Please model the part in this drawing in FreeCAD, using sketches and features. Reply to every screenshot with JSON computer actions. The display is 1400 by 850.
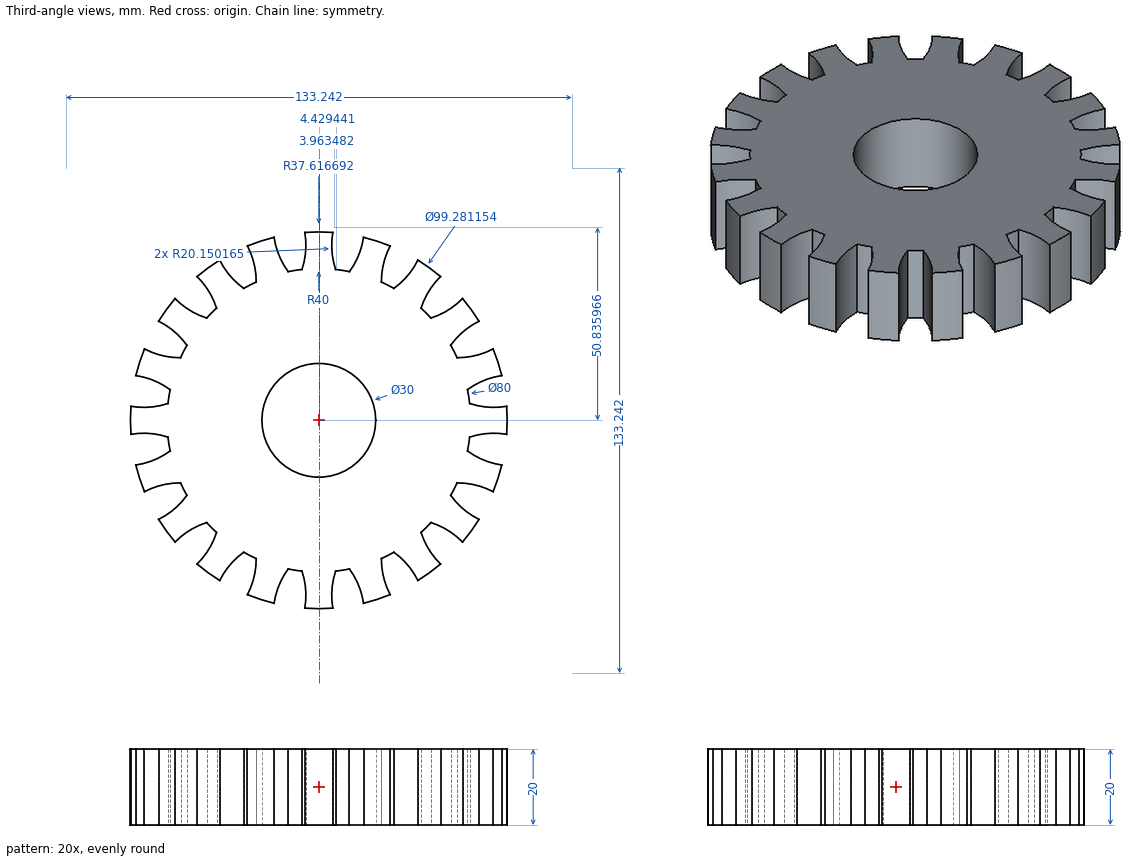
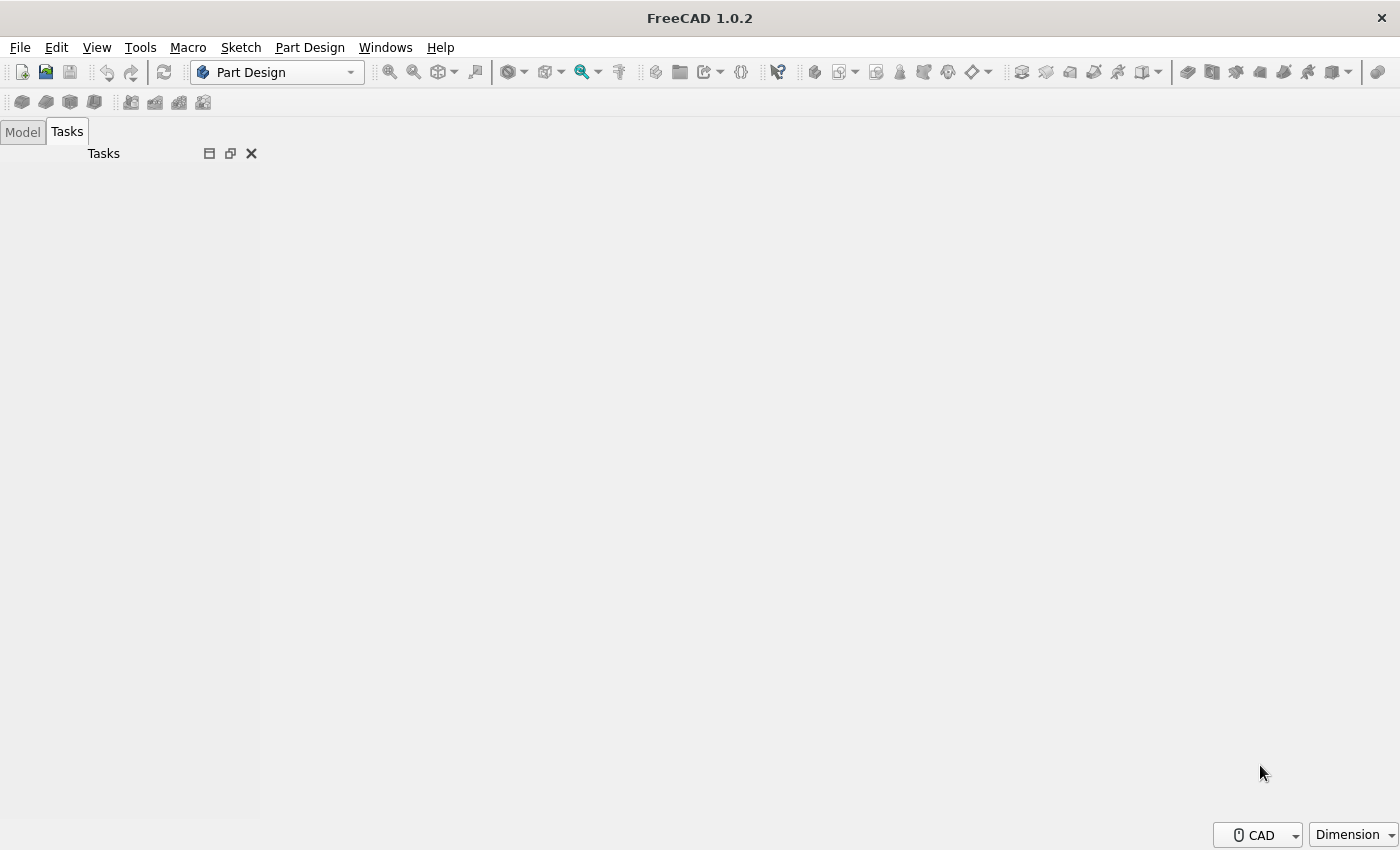
{"action": "left_click", "coordinate": [22, 72]}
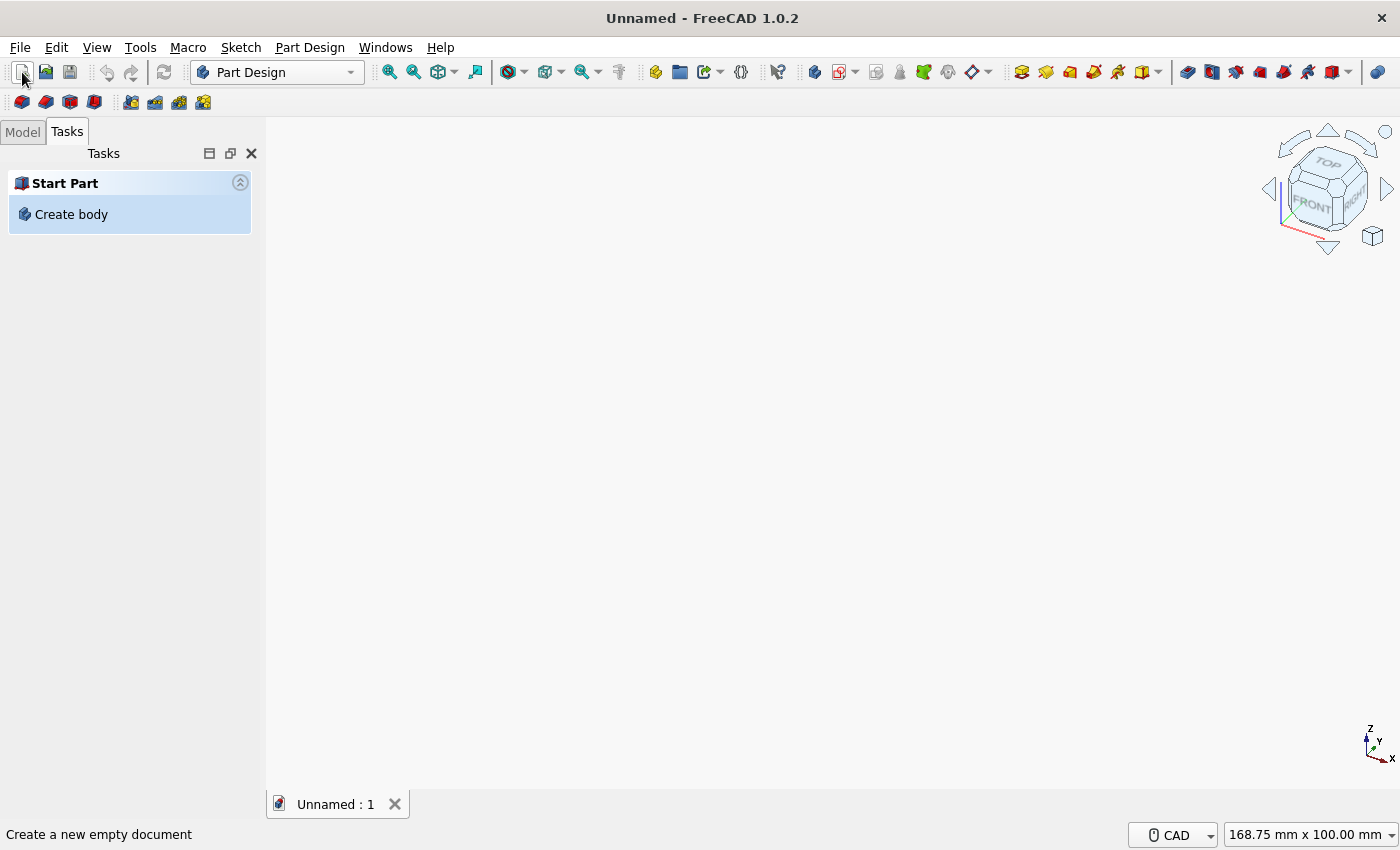
{"action": "left_click", "coordinate": [840, 72]}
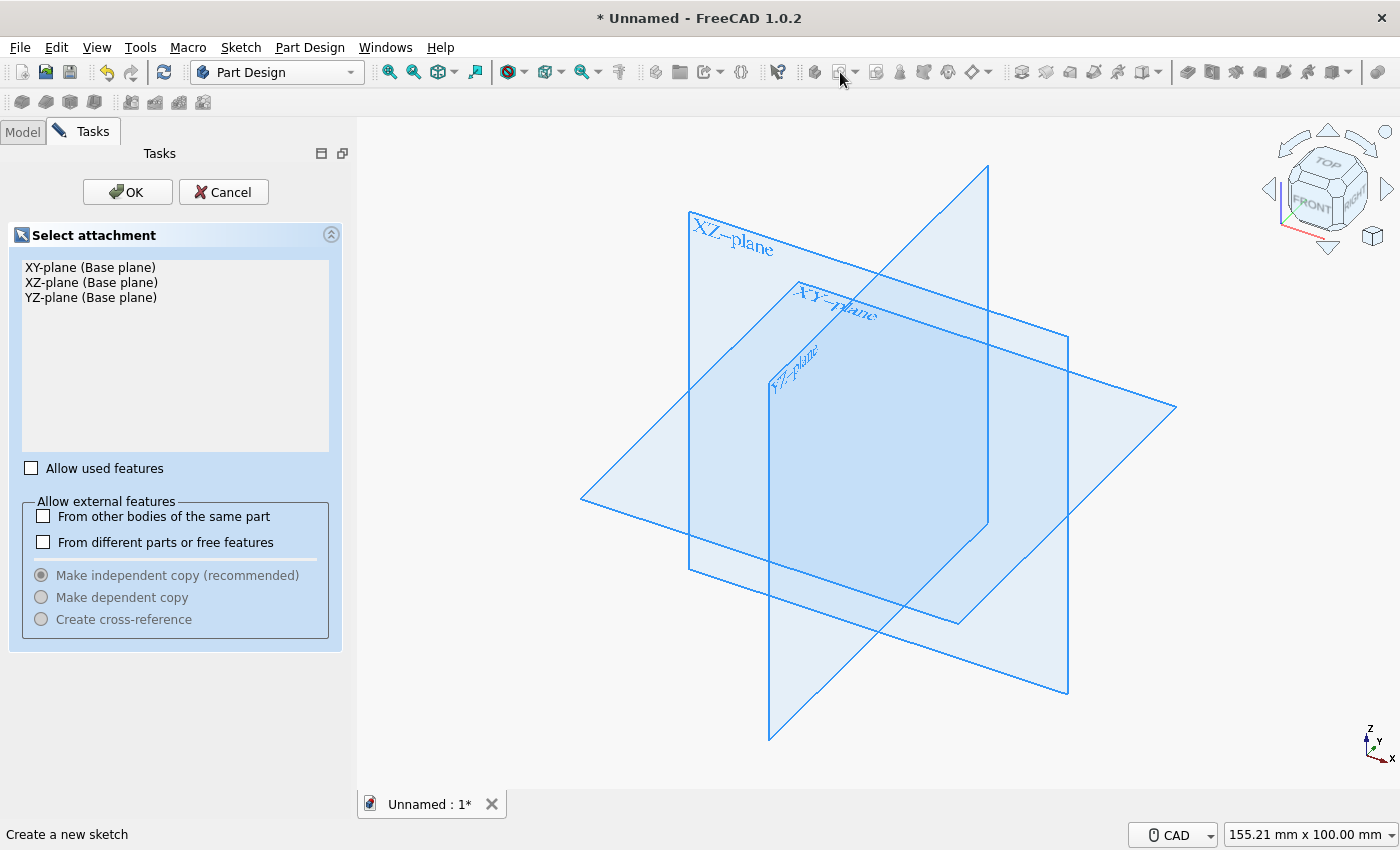
{"action": "left_click", "coordinate": [82, 268]}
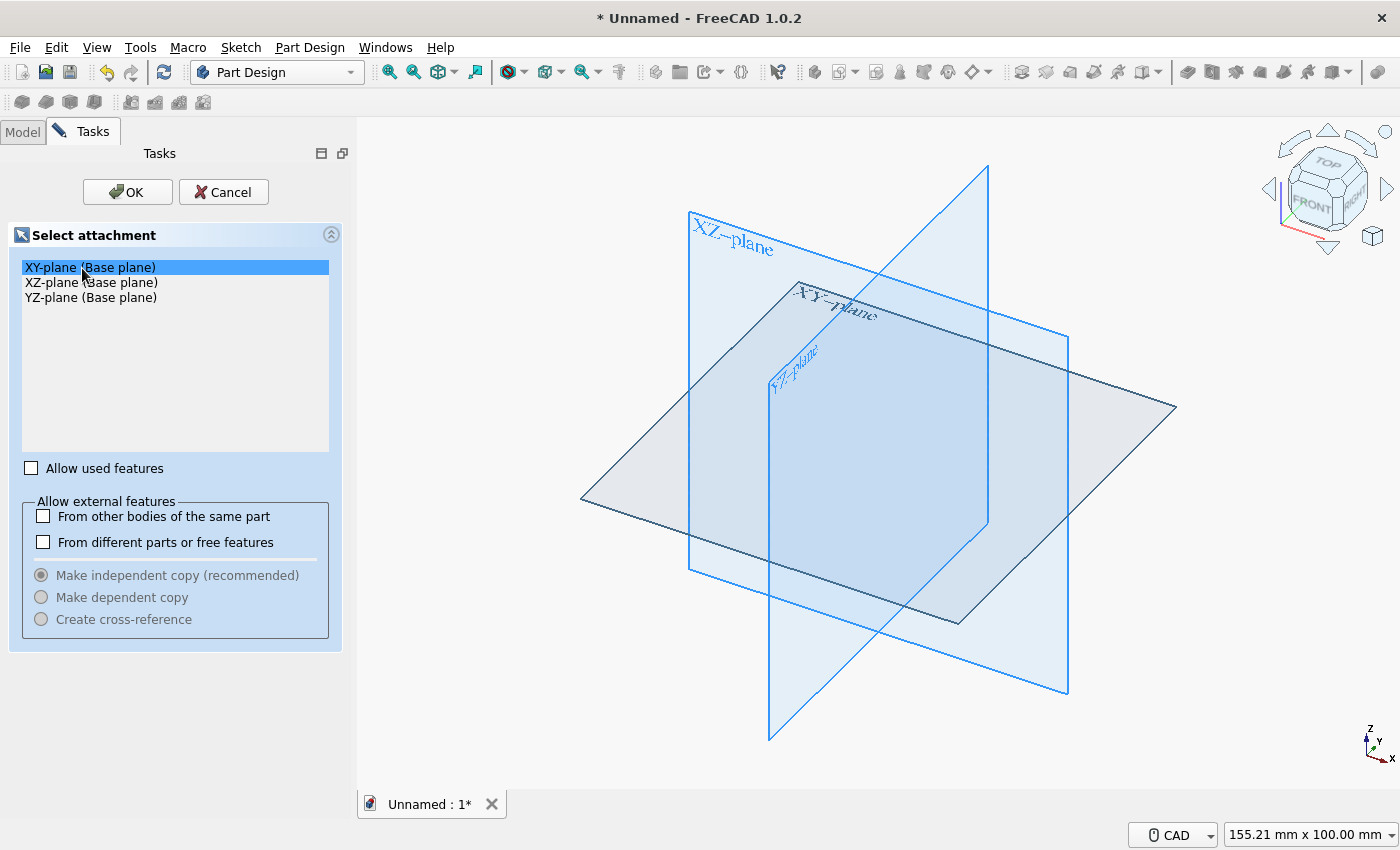
{"action": "left_click", "coordinate": [128, 192]}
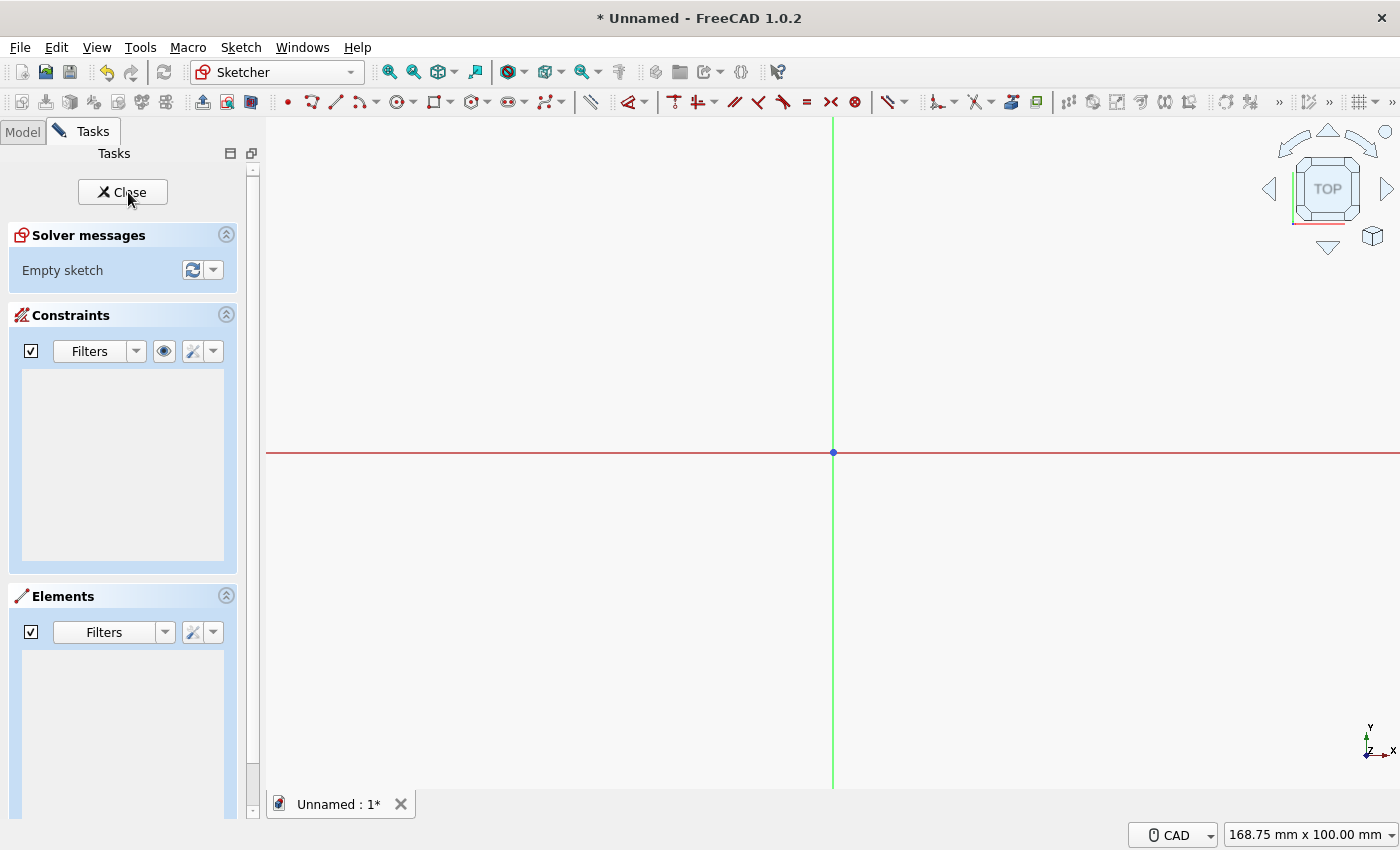
{"action": "left_click", "coordinate": [398, 102]}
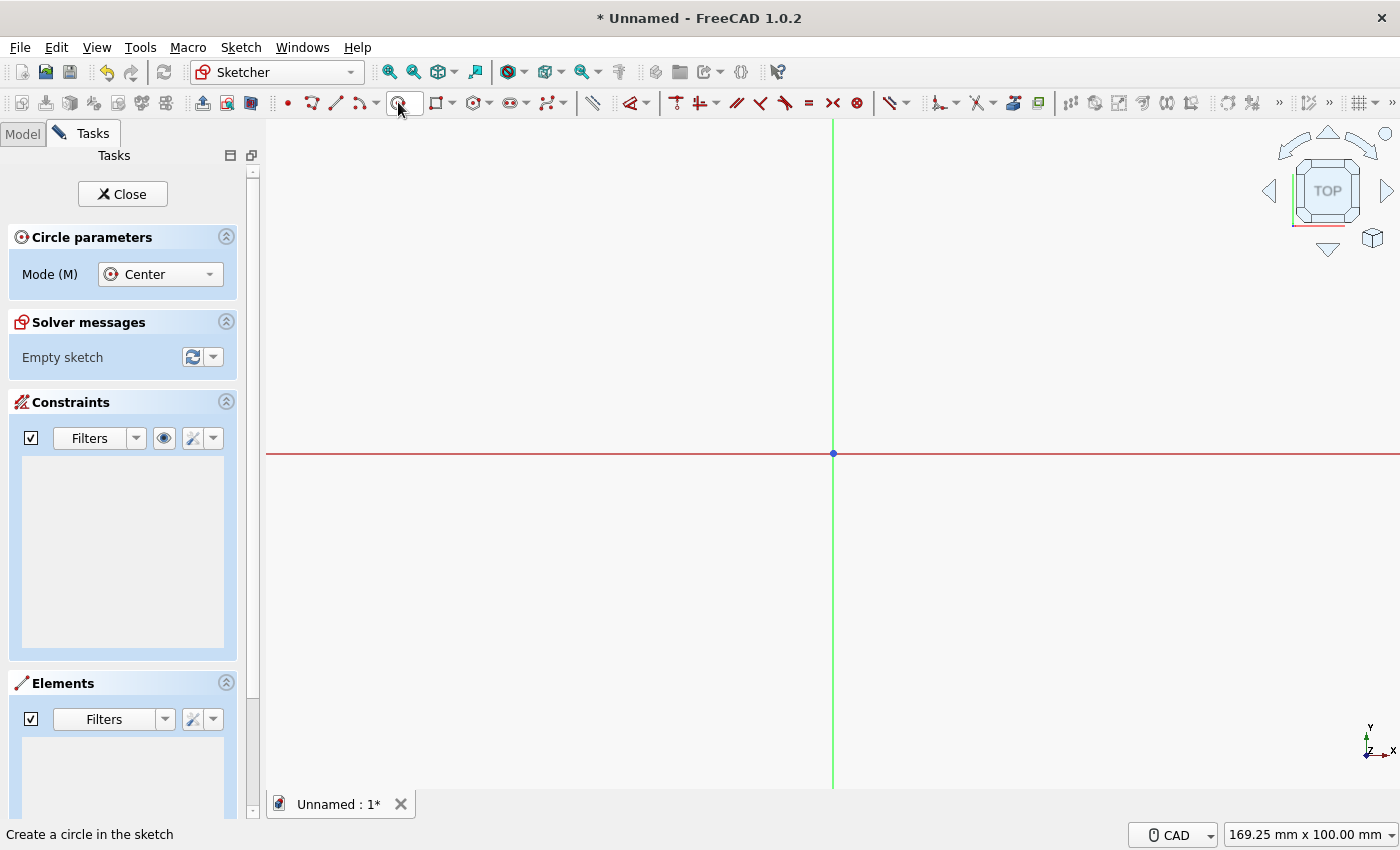
{"action": "left_click", "coordinate": [833, 454]}
{"action": "left_click", "coordinate": [1023, 264]}
{"action": "key", "text": "Escape"}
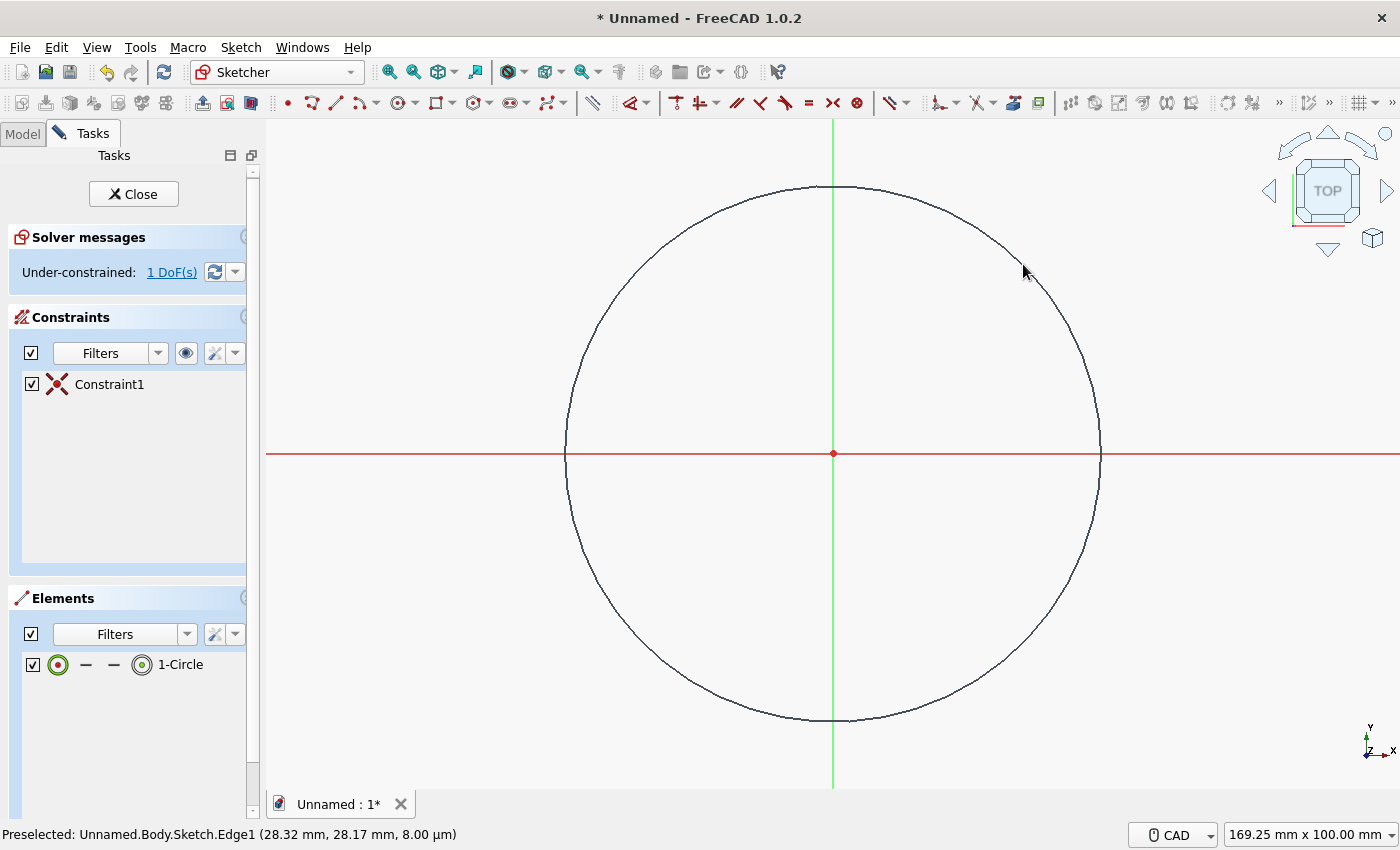
{"action": "key", "text": "d"}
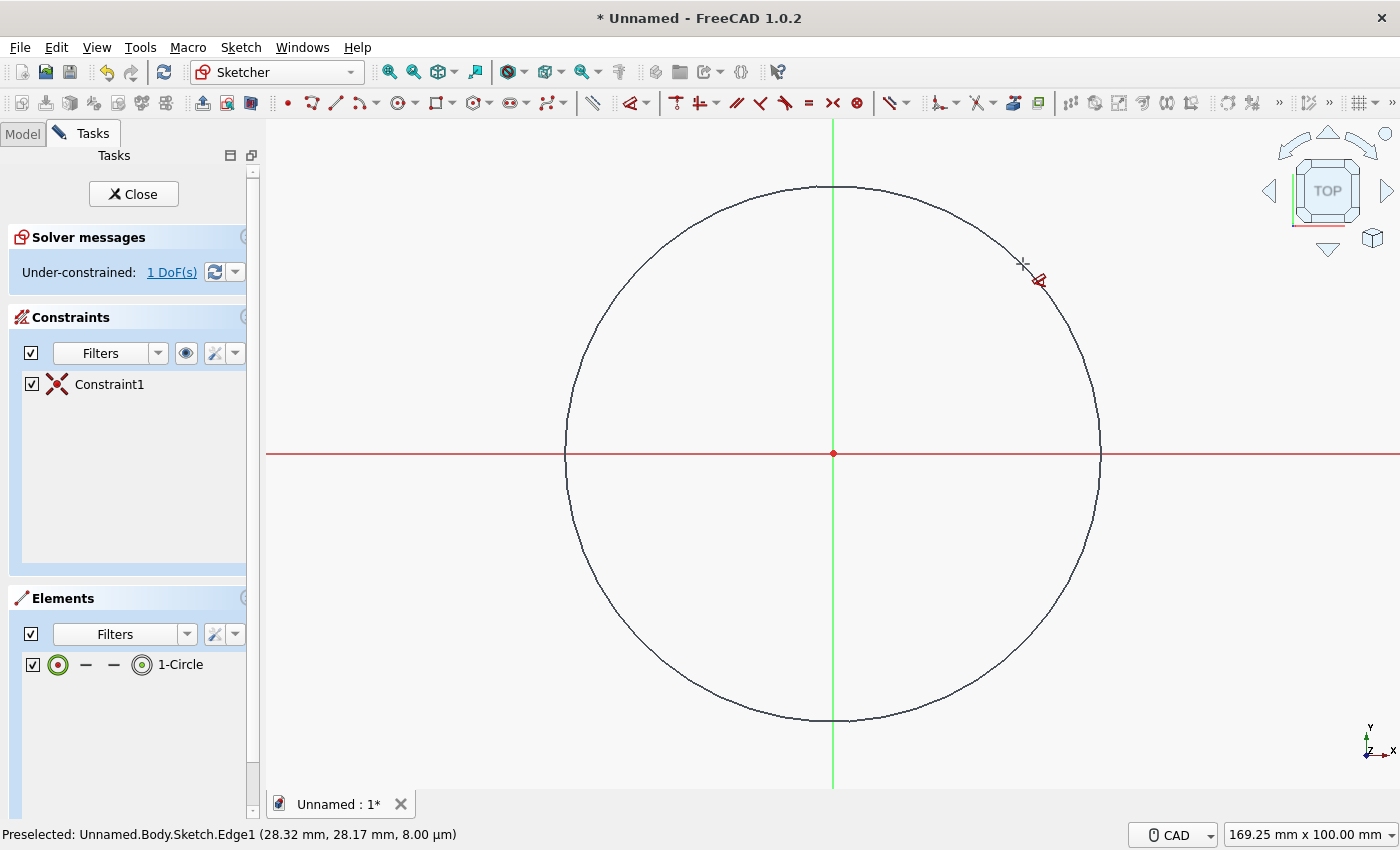
{"action": "left_click", "coordinate": [1022, 264]}
{"action": "left_click", "coordinate": [1045, 241]}